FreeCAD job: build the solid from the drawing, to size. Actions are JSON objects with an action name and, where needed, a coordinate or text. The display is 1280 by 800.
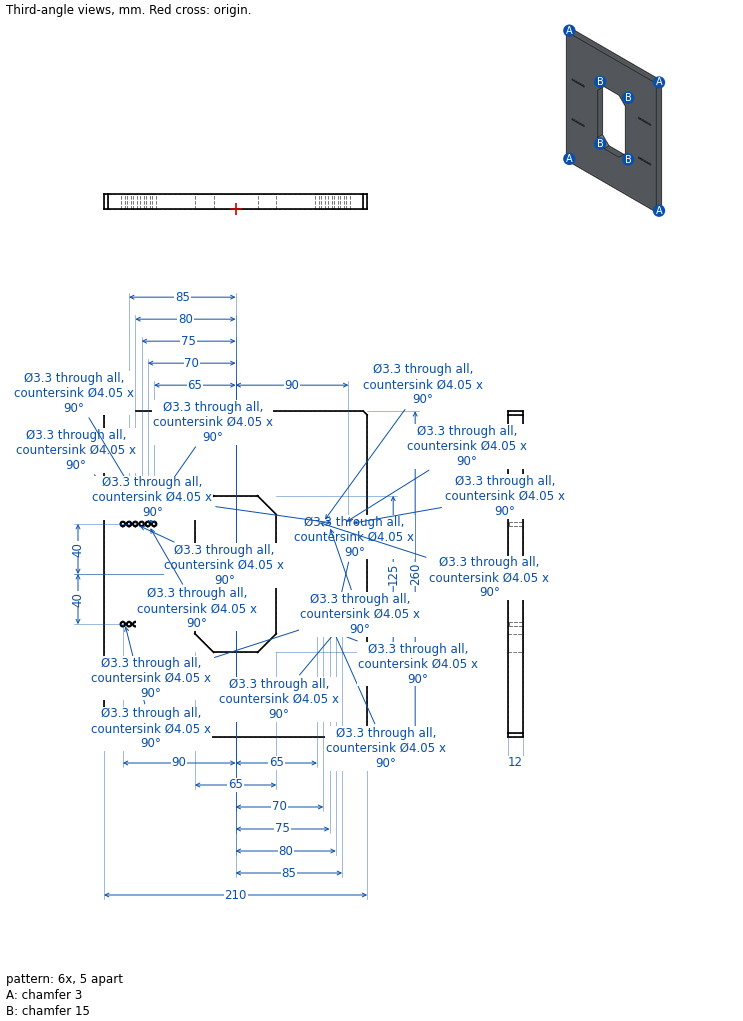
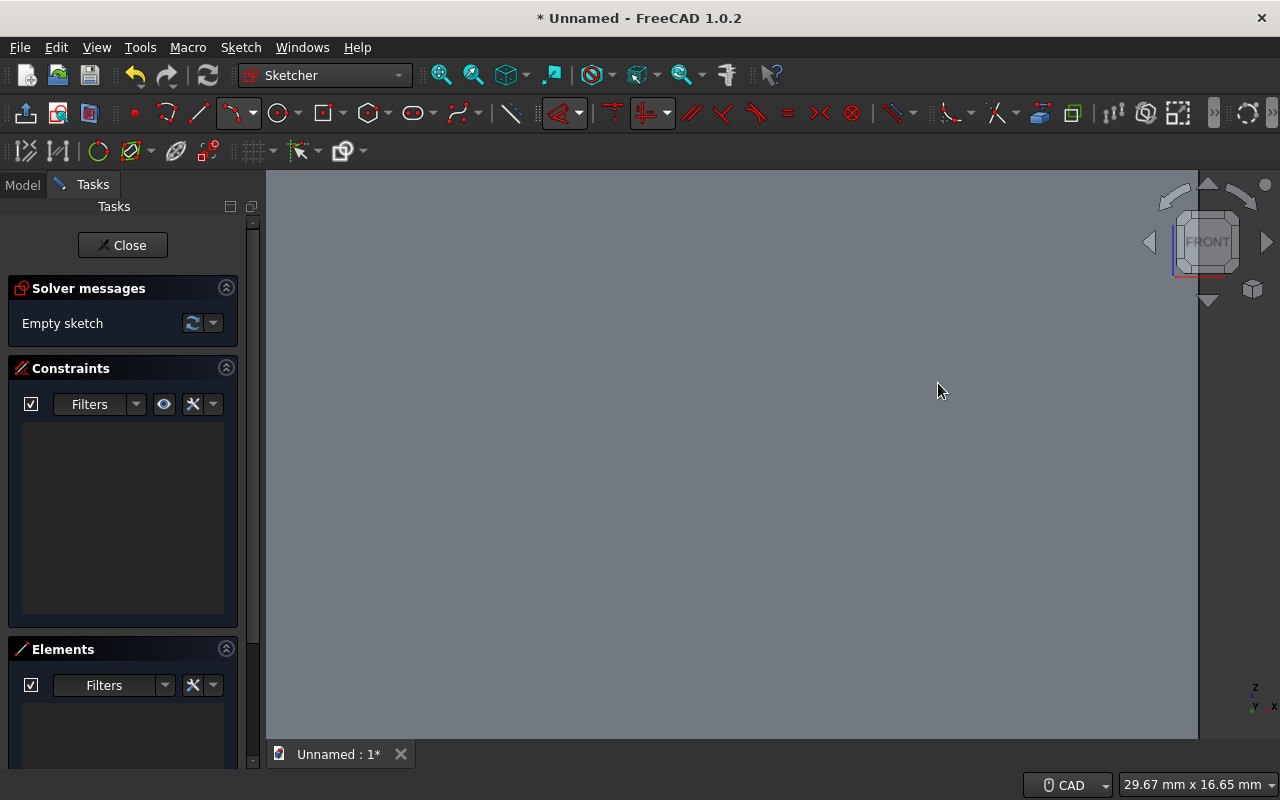
{"action": "scroll", "coordinate": [679, 441], "scroll_direction": "up", "scroll_amount": 6}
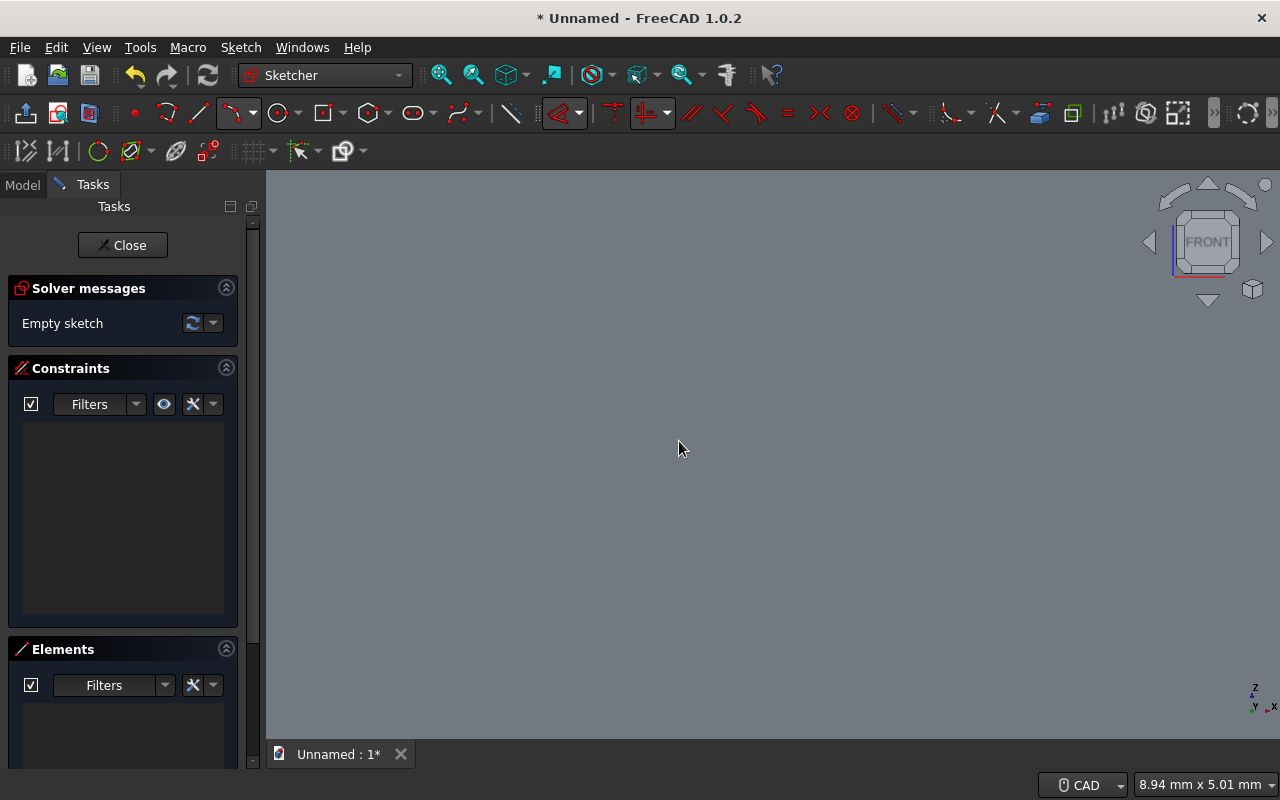
{"action": "left_click", "coordinate": [278, 114]}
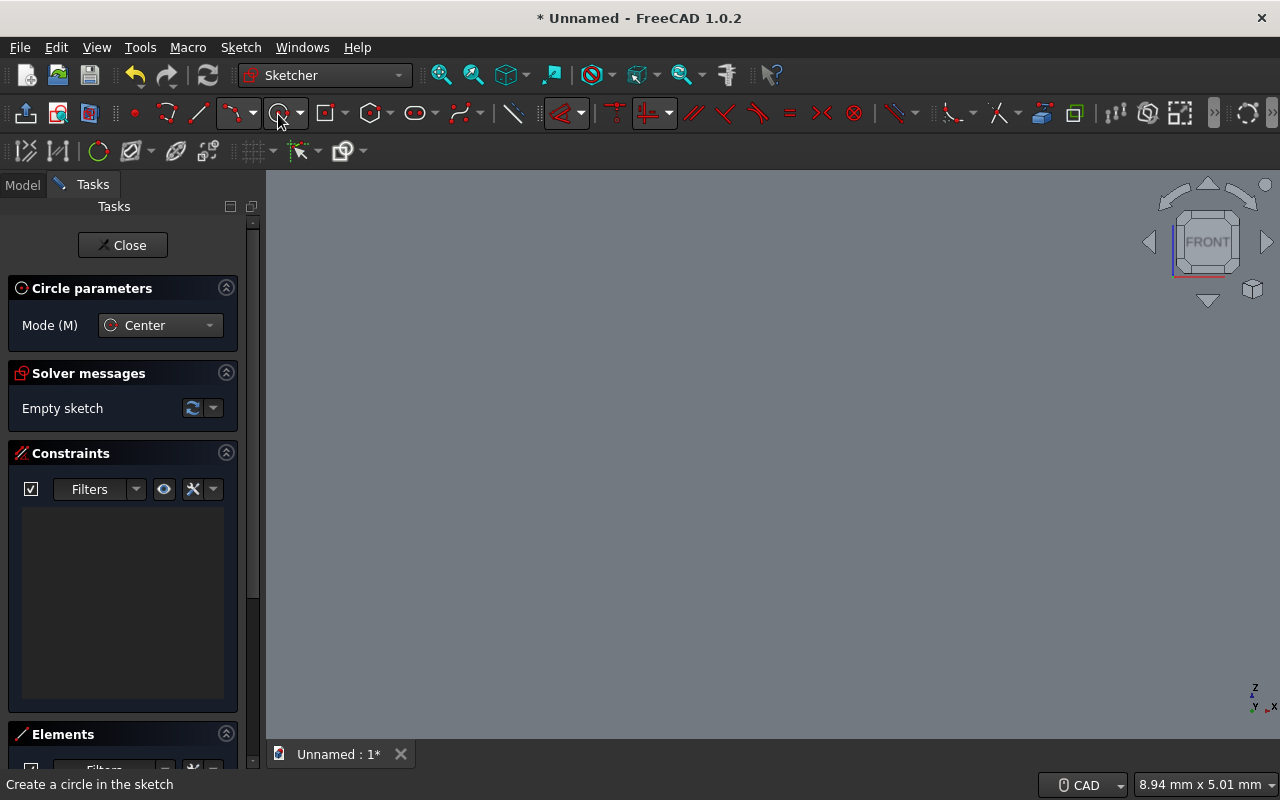
{"action": "left_click", "coordinate": [704, 453]}
{"action": "mouse_move", "coordinate": [836, 321]}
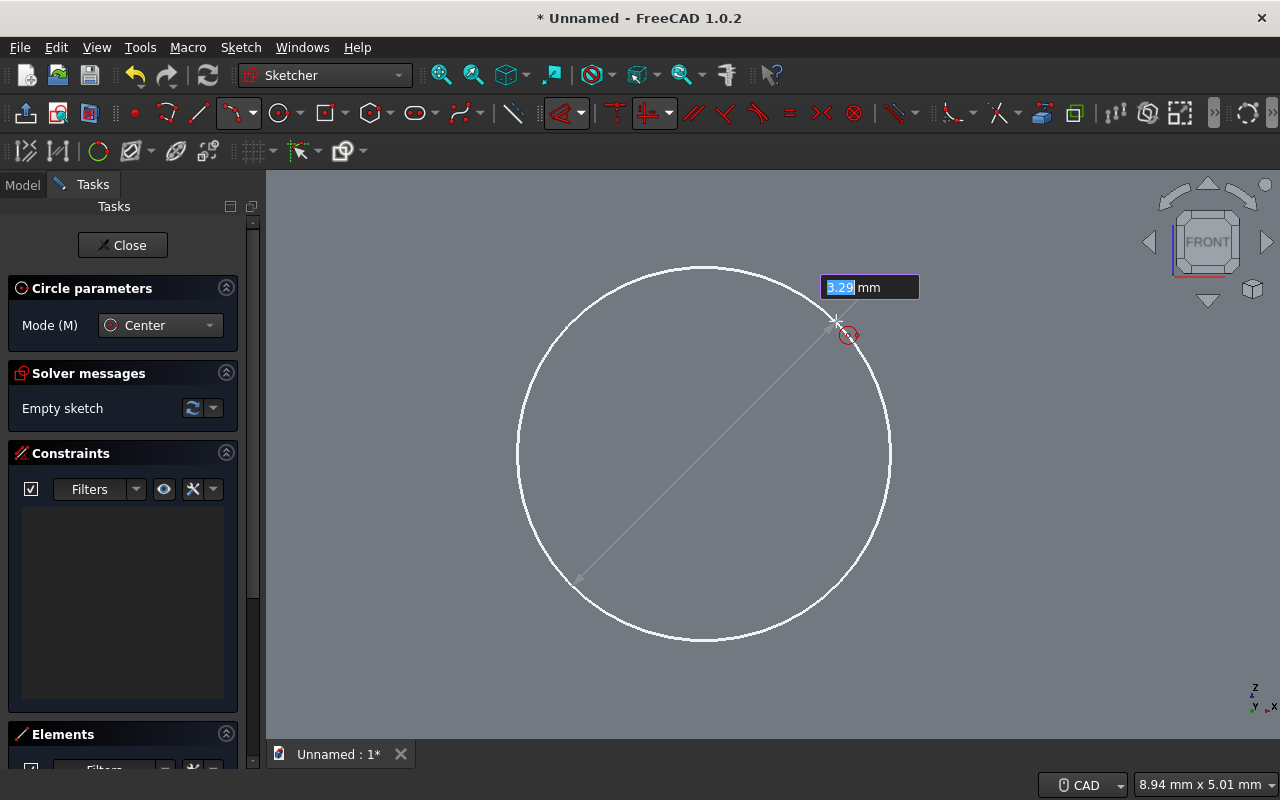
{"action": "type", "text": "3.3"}
{"action": "key", "text": "Return"}
{"action": "key", "text": "Escape"}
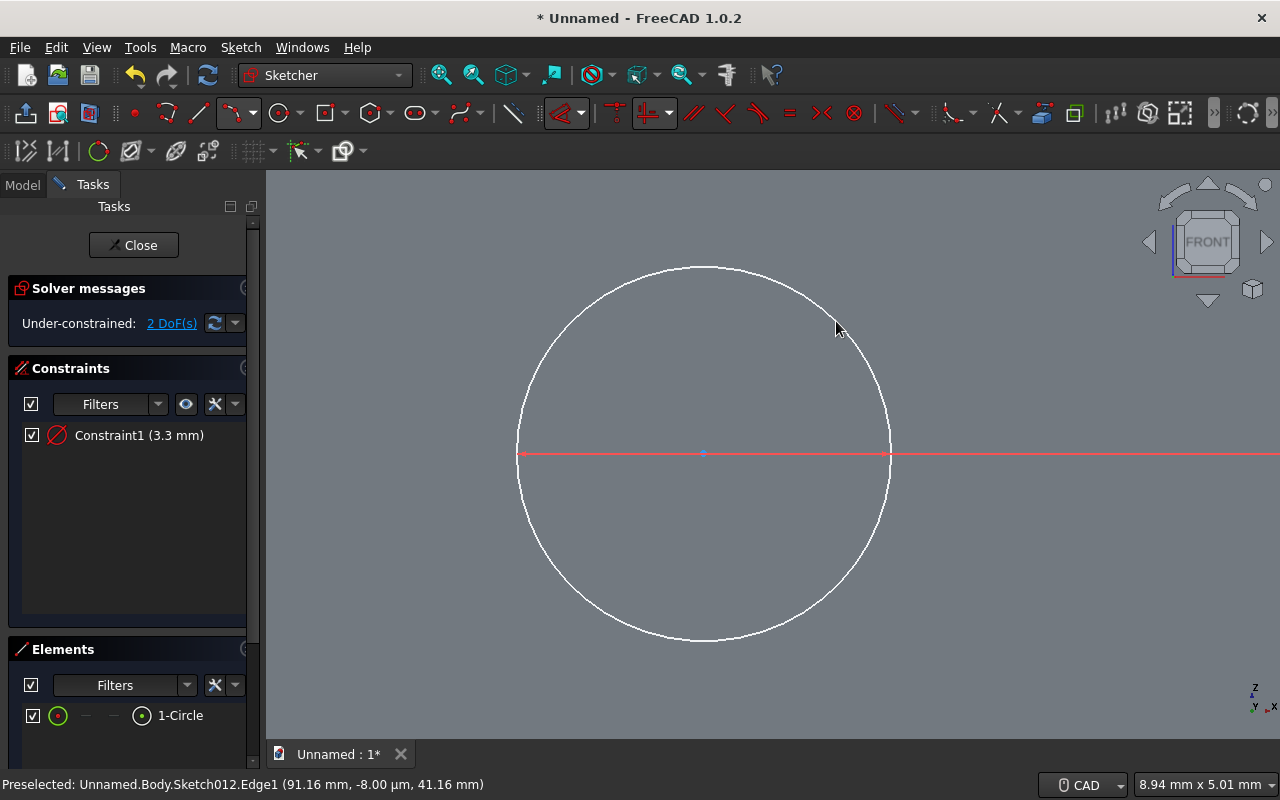
{"action": "left_click", "coordinate": [704, 454]}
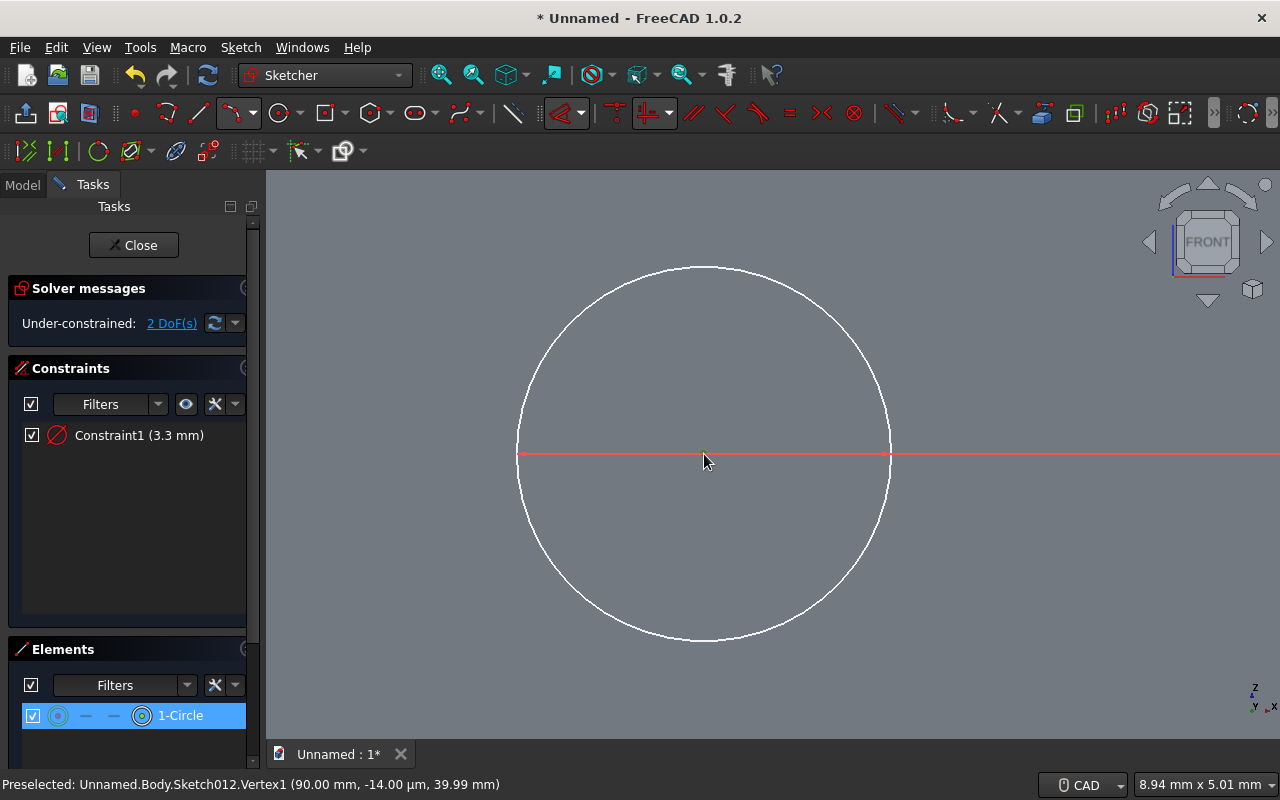
{"action": "left_click", "coordinate": [584, 114]}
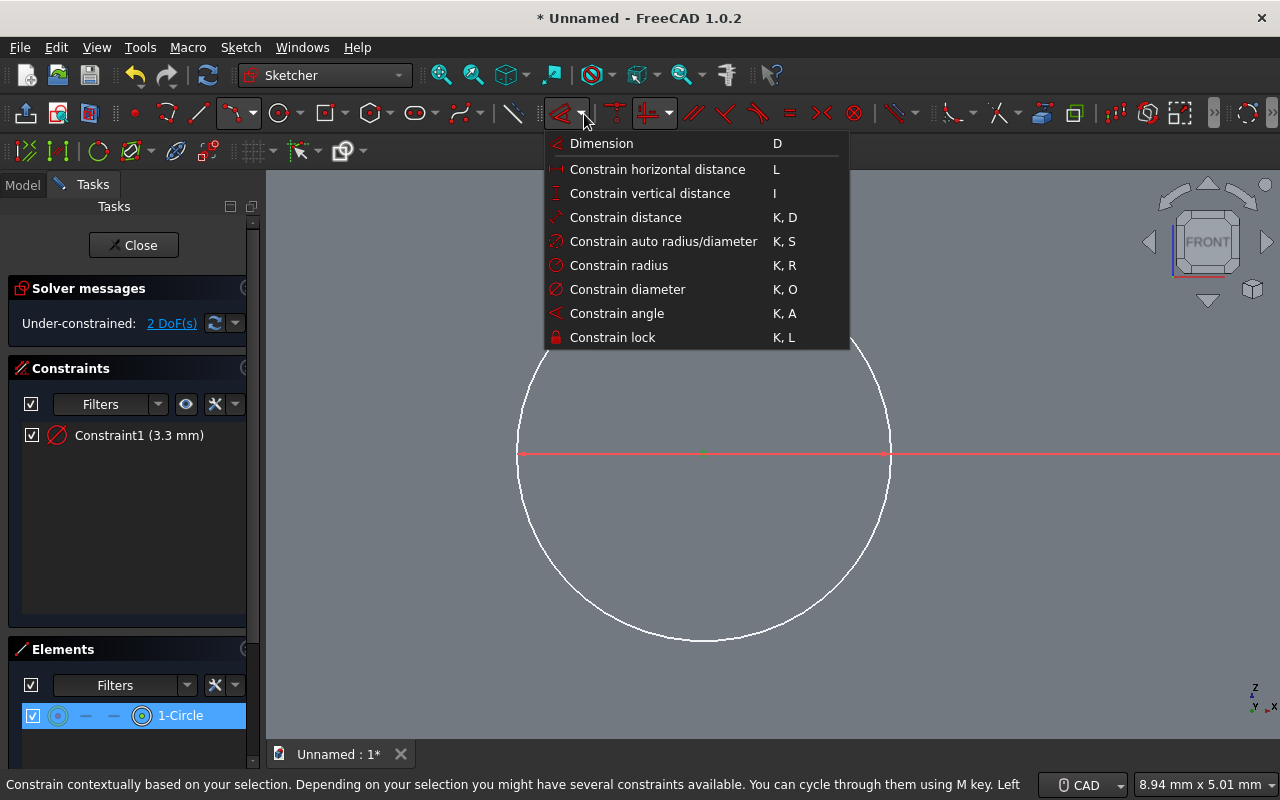
{"action": "left_click", "coordinate": [697, 169]}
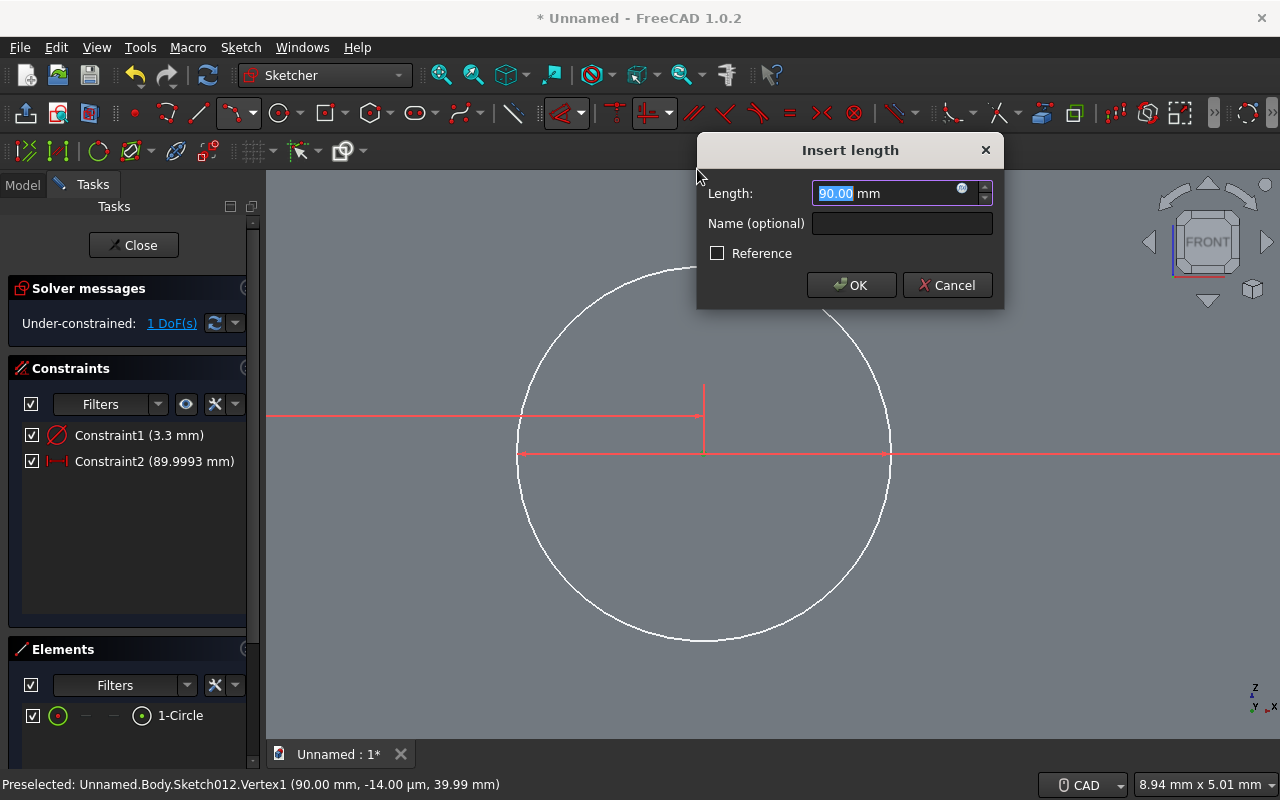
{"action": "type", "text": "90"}
{"action": "key", "text": "Return"}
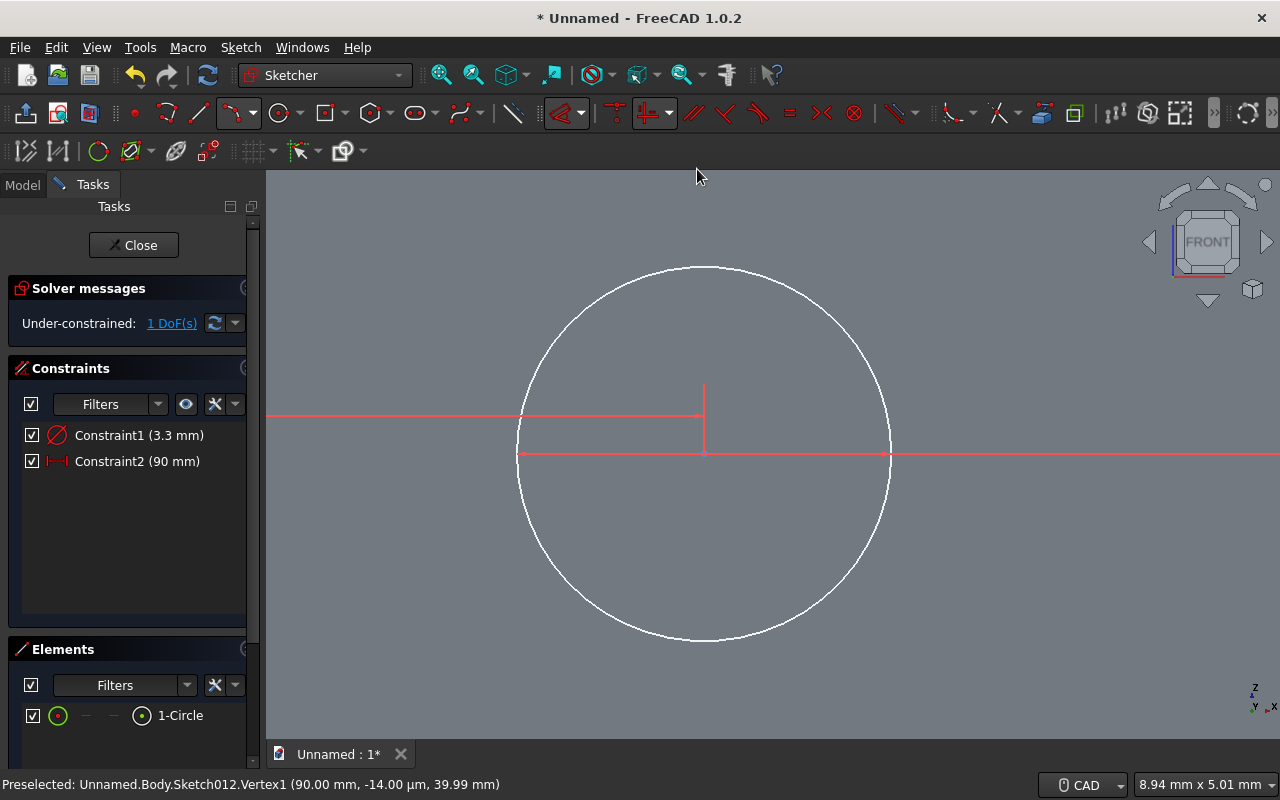
{"action": "left_click", "coordinate": [704, 454]}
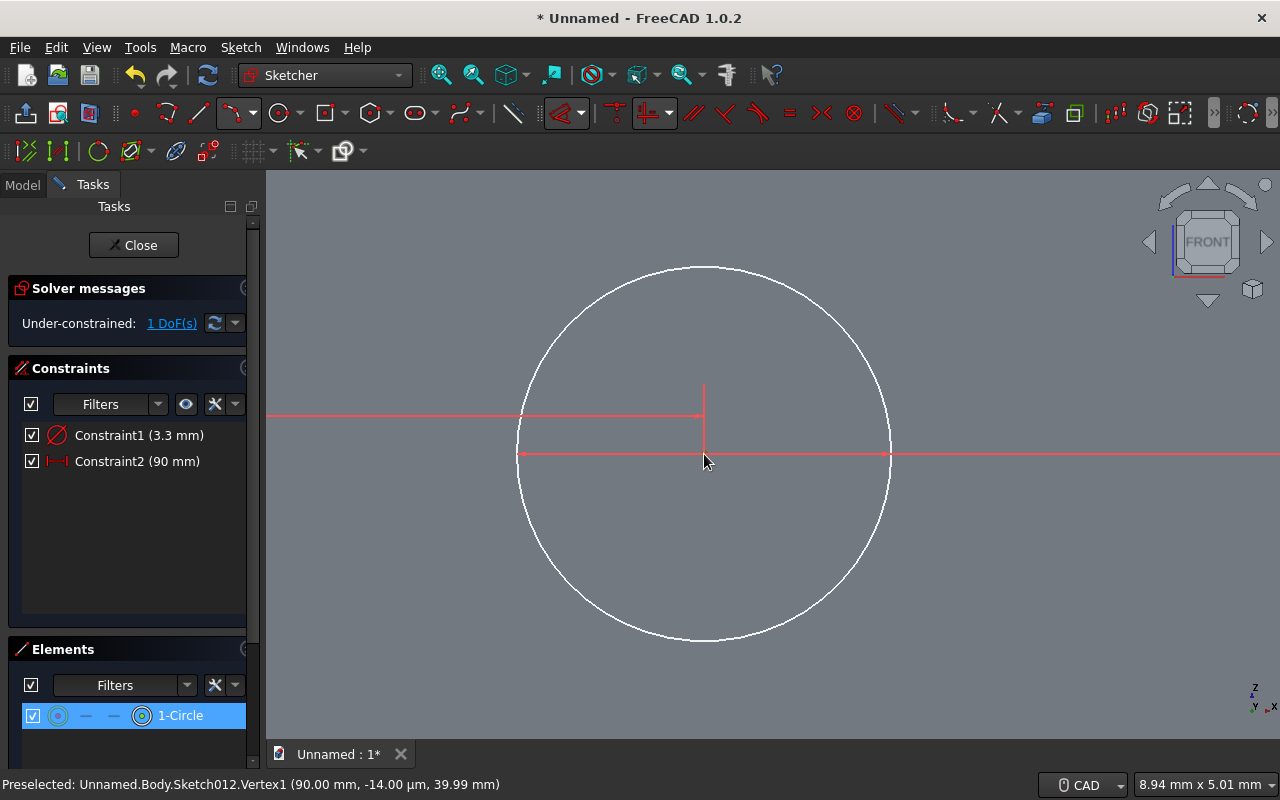
{"action": "key", "text": "i"}